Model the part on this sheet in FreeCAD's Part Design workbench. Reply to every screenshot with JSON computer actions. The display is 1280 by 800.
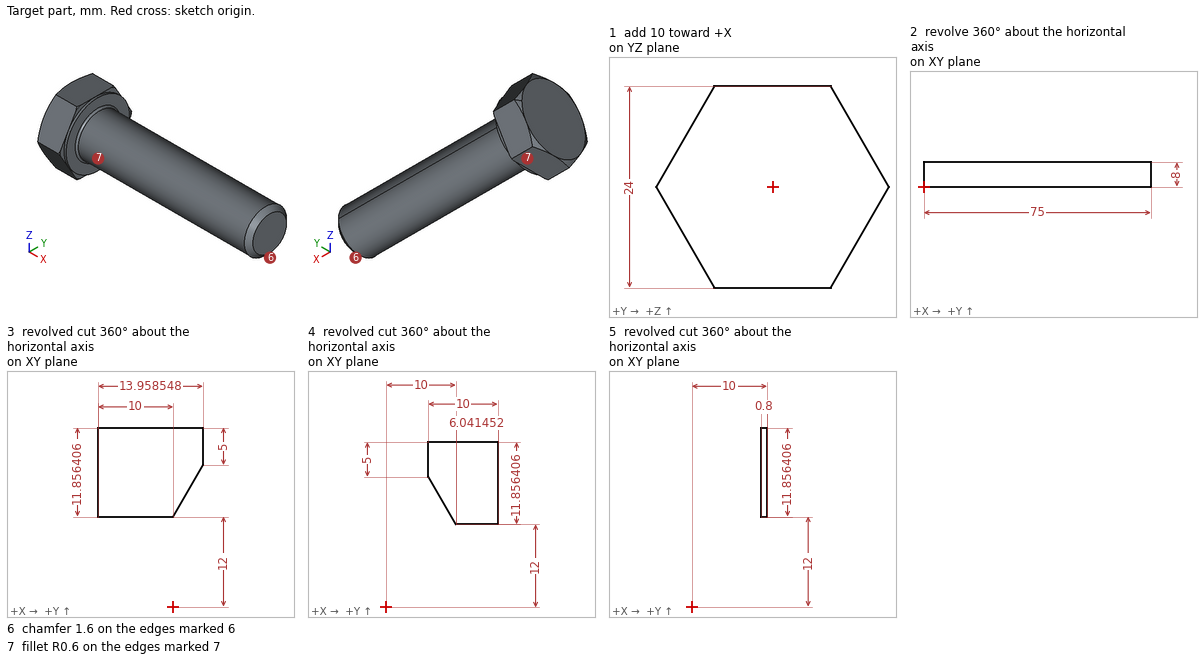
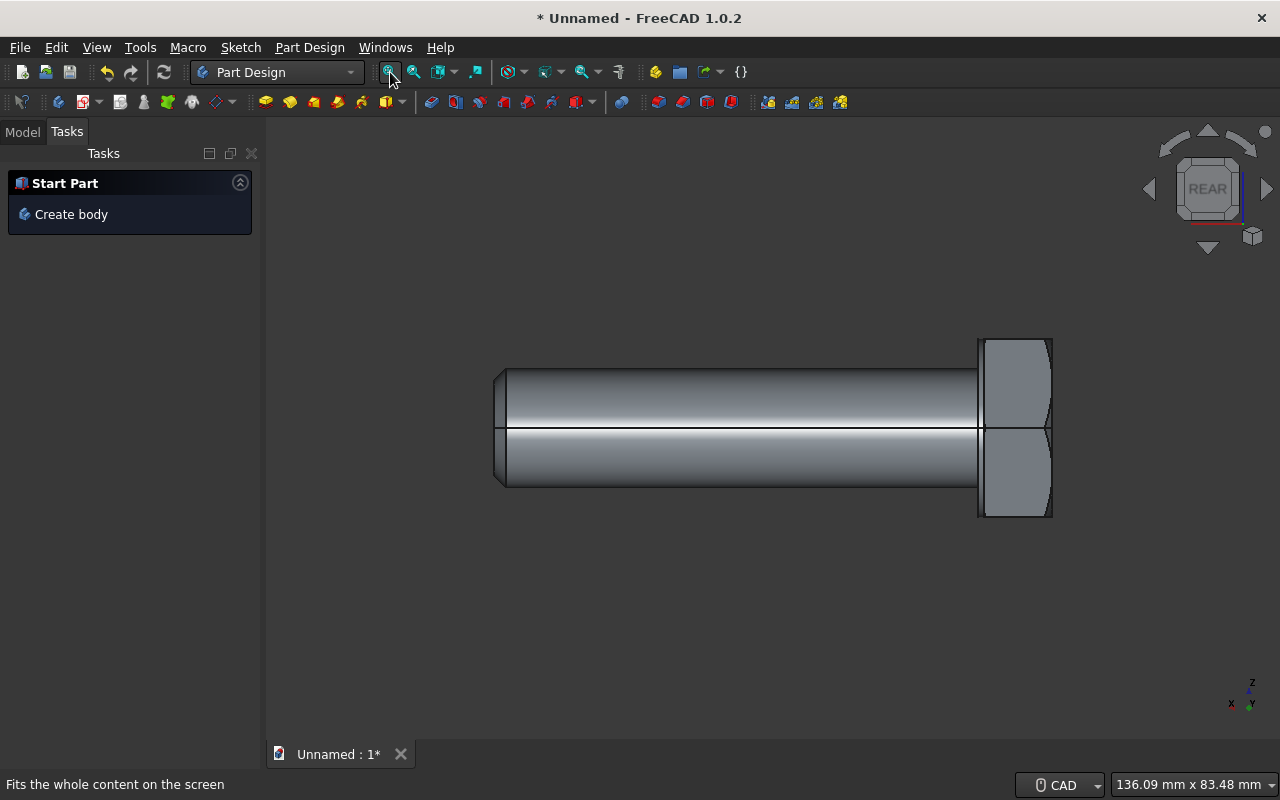
{"action": "key", "text": "6"}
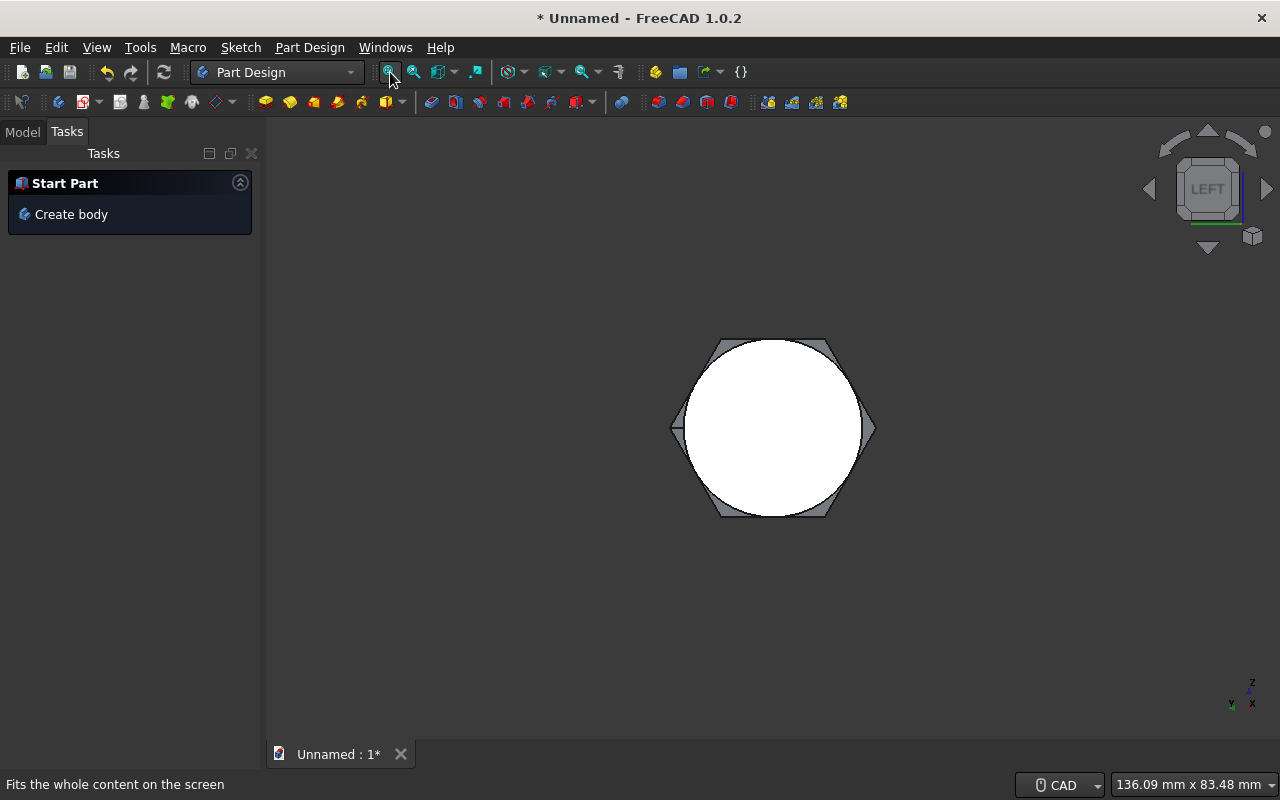
{"action": "left_click", "coordinate": [390, 72]}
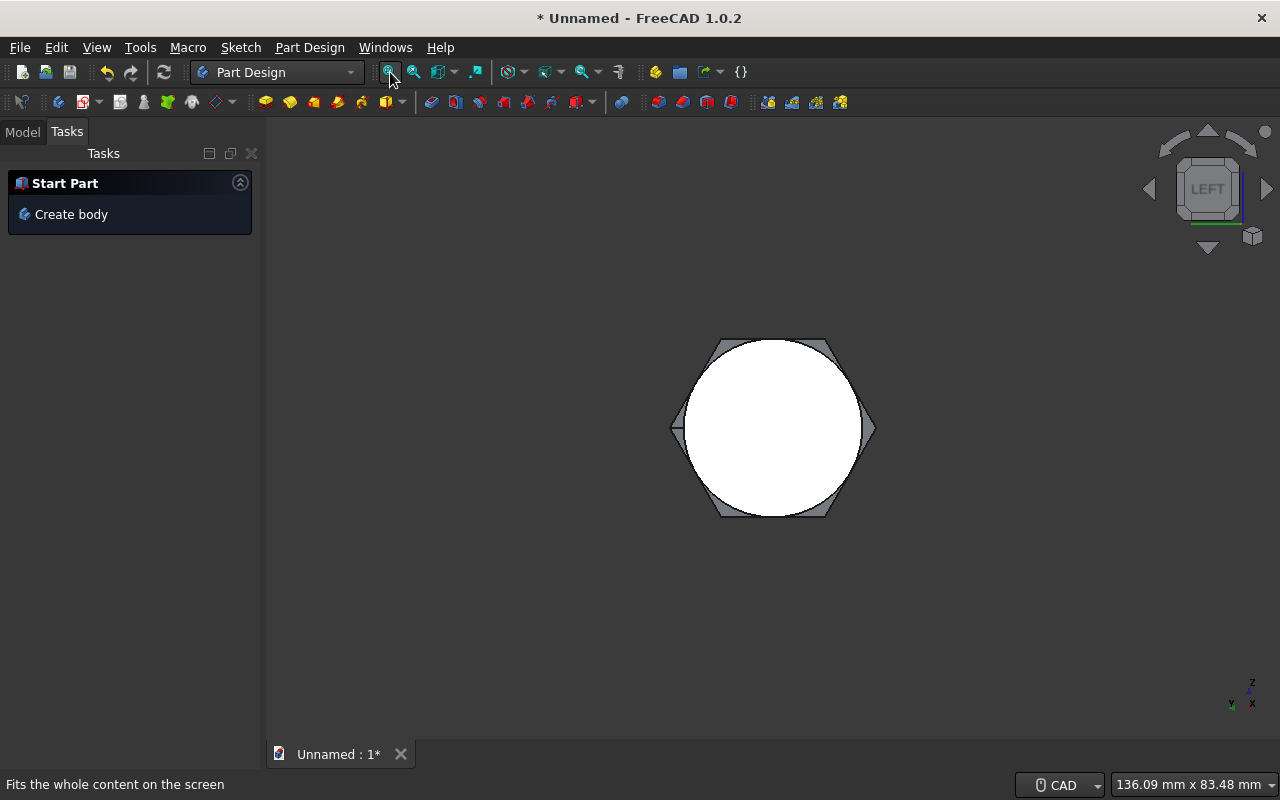
{"action": "key", "text": "v 3"}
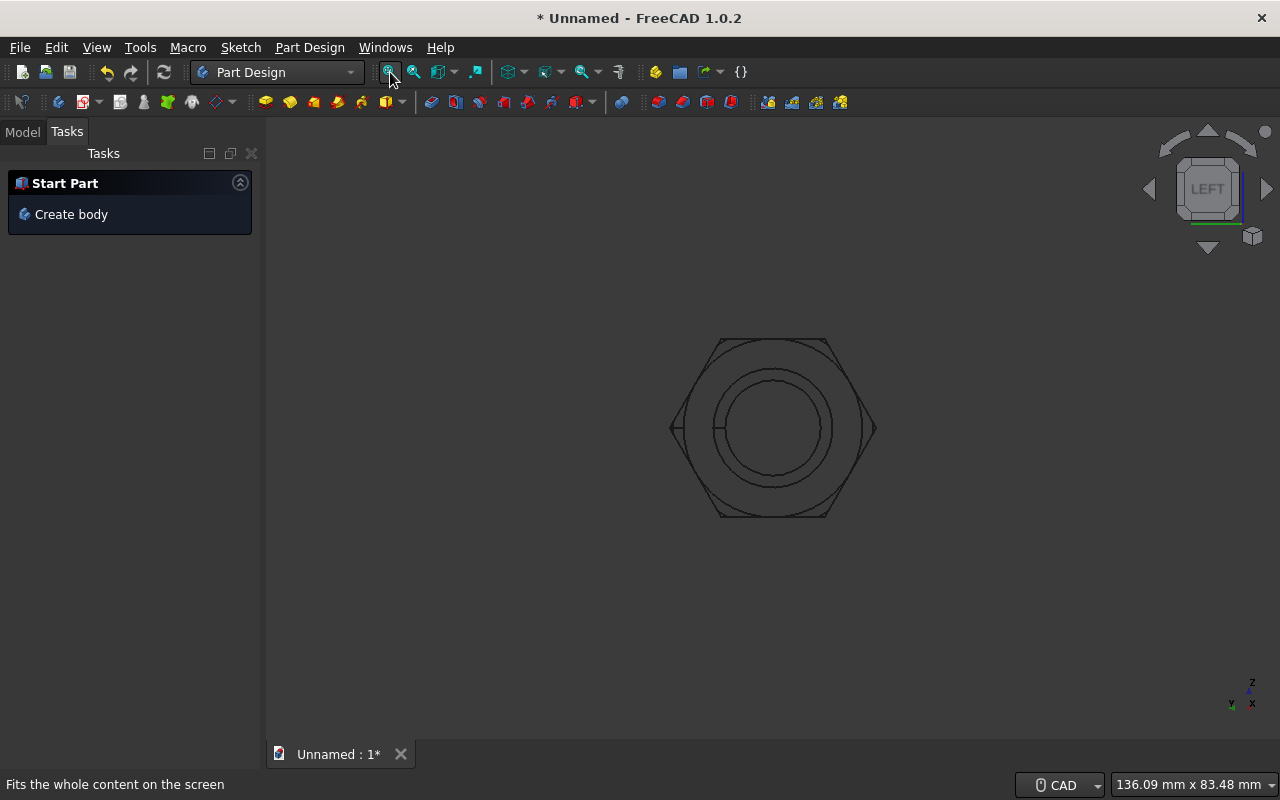
{"action": "key", "text": "0"}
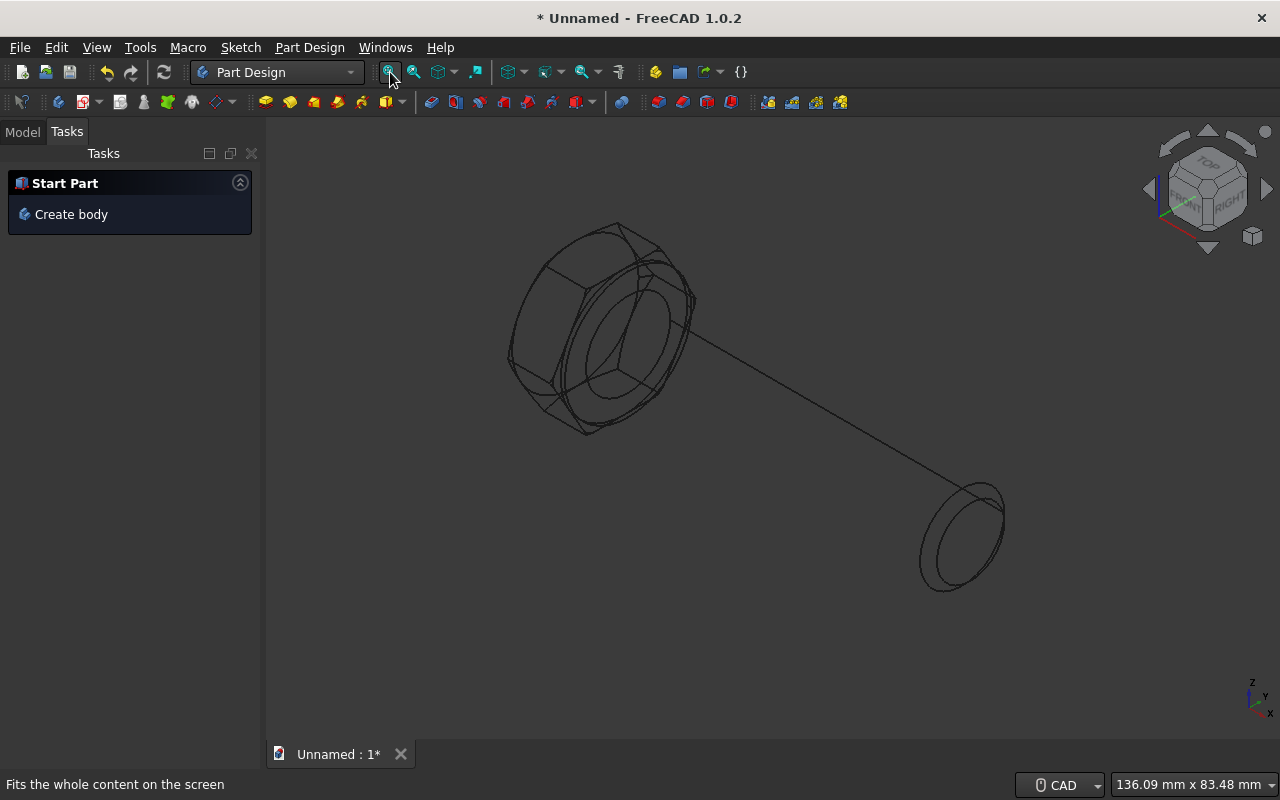
{"action": "left_click", "coordinate": [586, 368]}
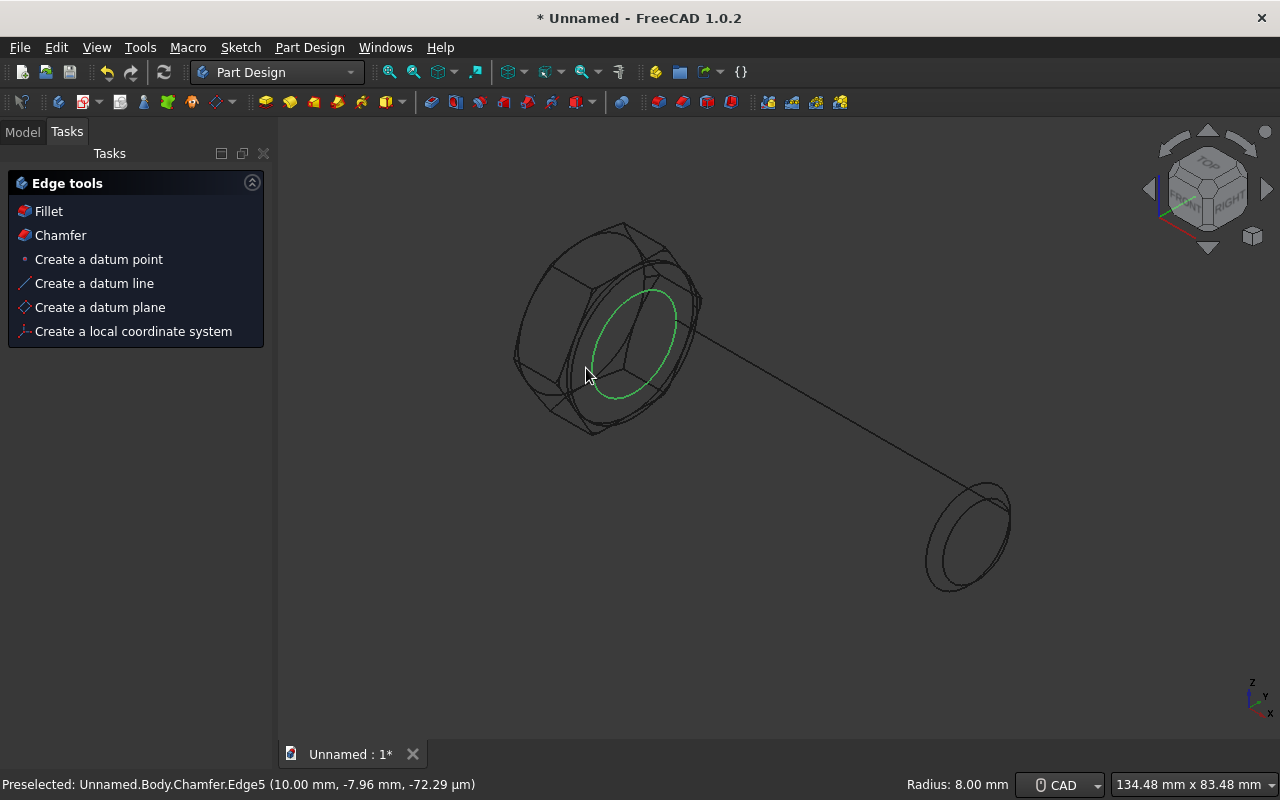
{"action": "key", "text": "v 1"}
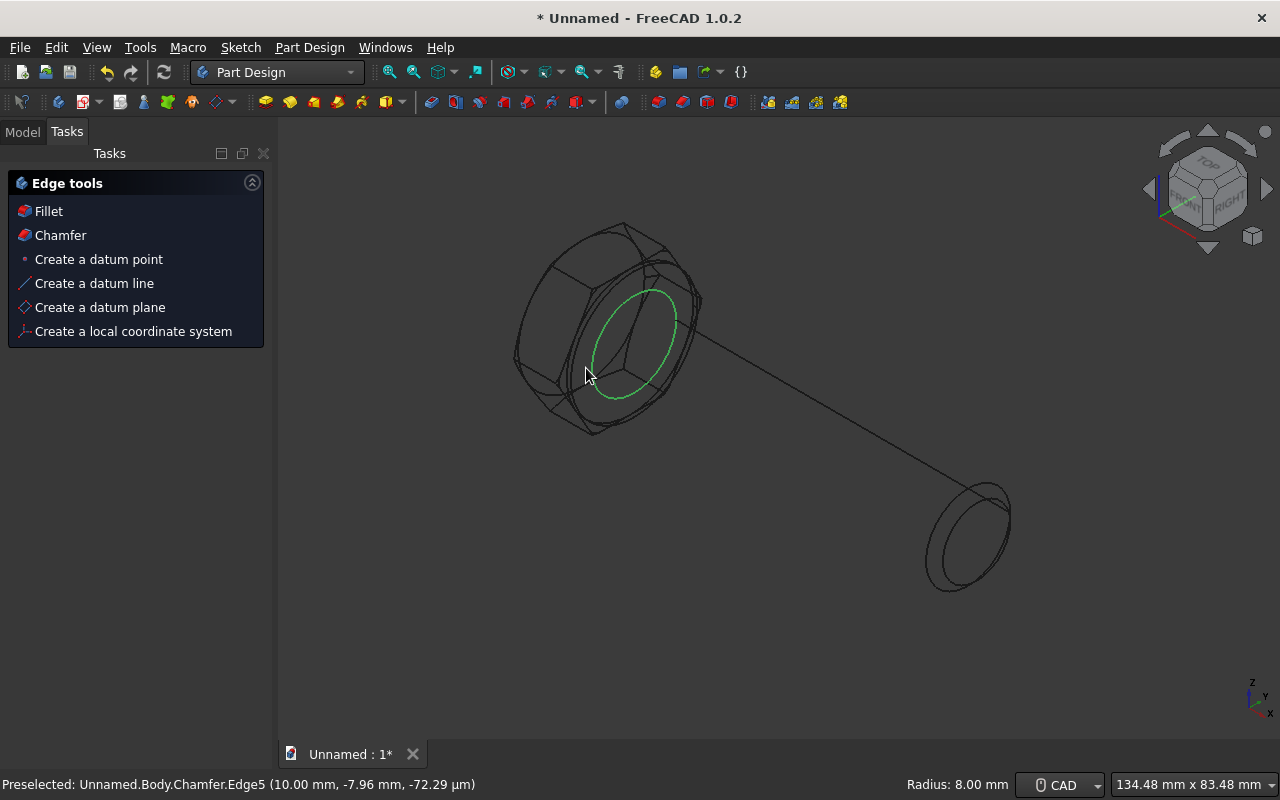
{"action": "left_click", "coordinate": [660, 102]}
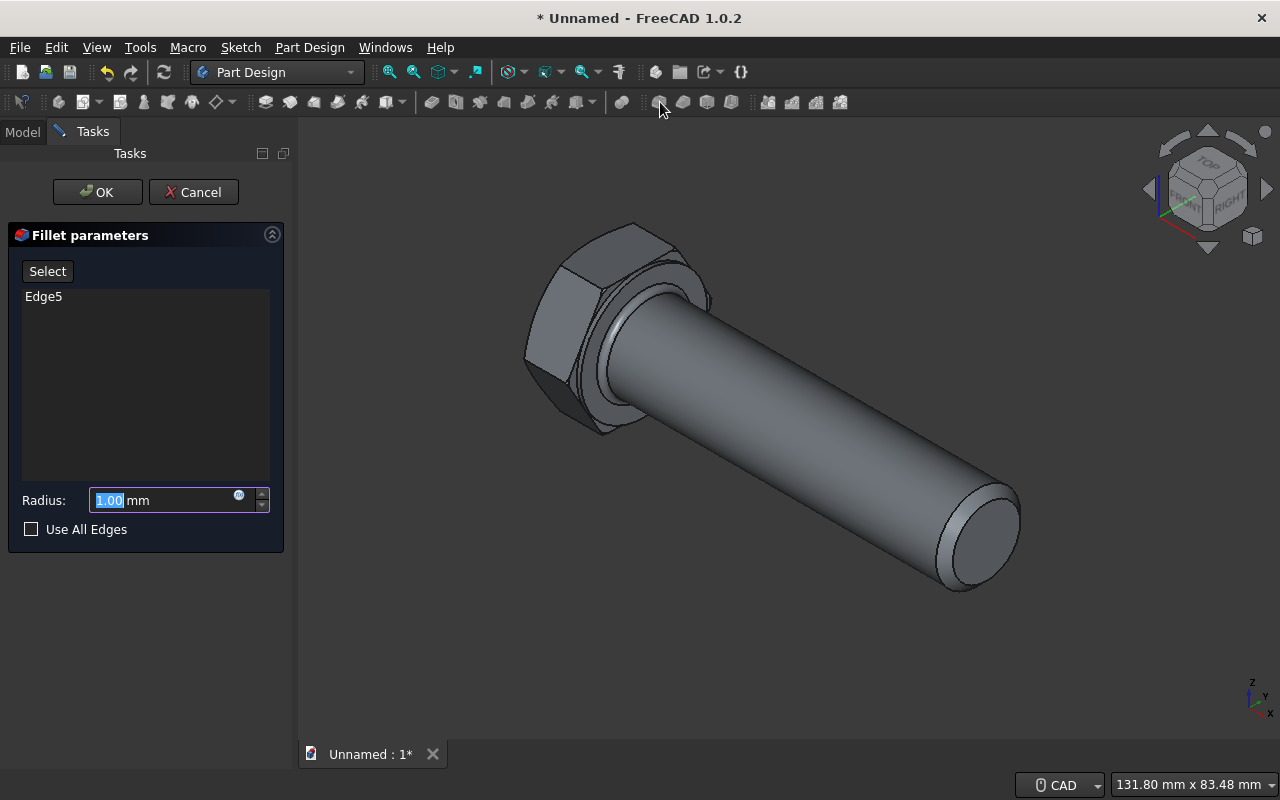
{"action": "type", "text": "0.6"}
{"action": "key", "text": "Tab"}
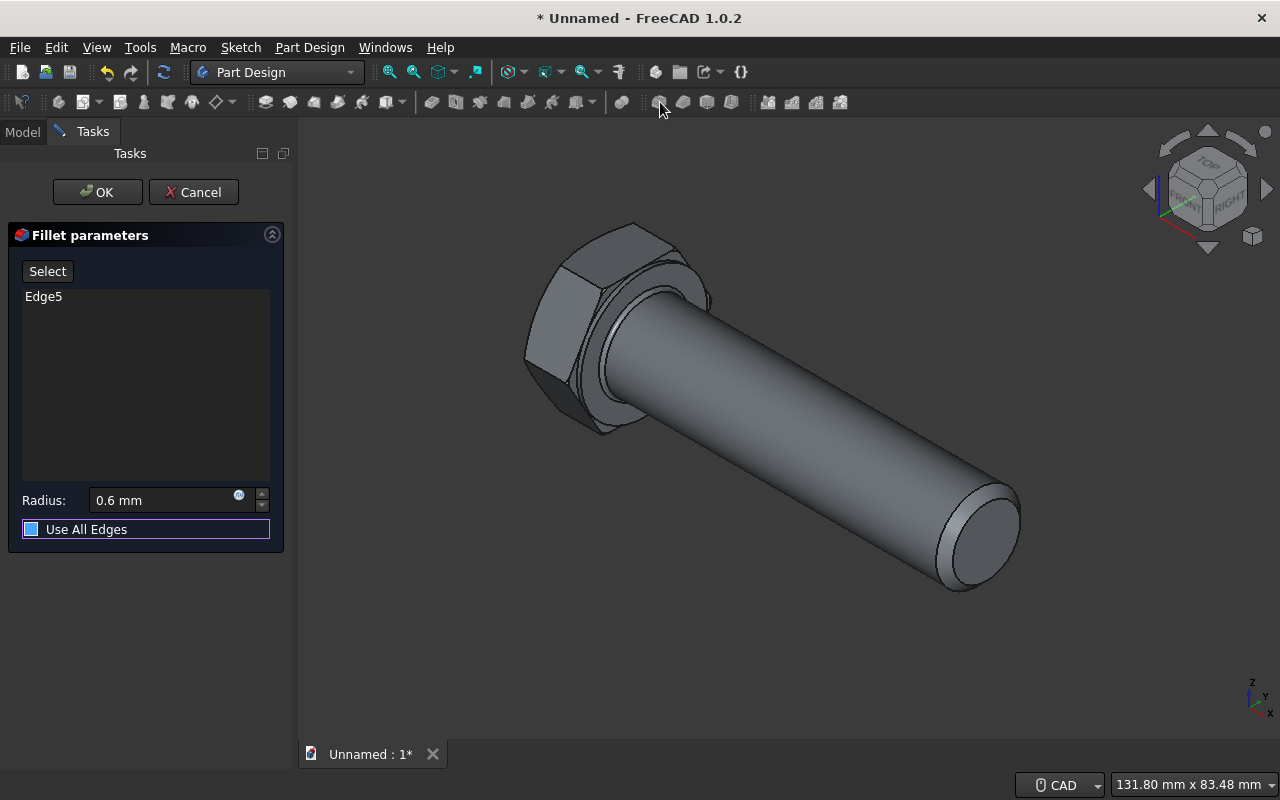
{"action": "left_click", "coordinate": [98, 192]}